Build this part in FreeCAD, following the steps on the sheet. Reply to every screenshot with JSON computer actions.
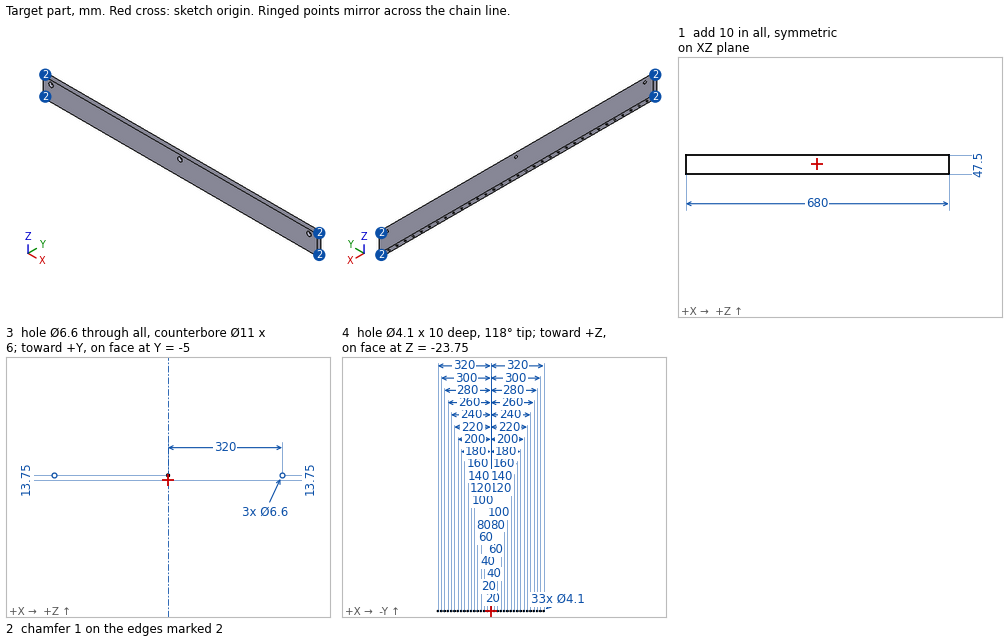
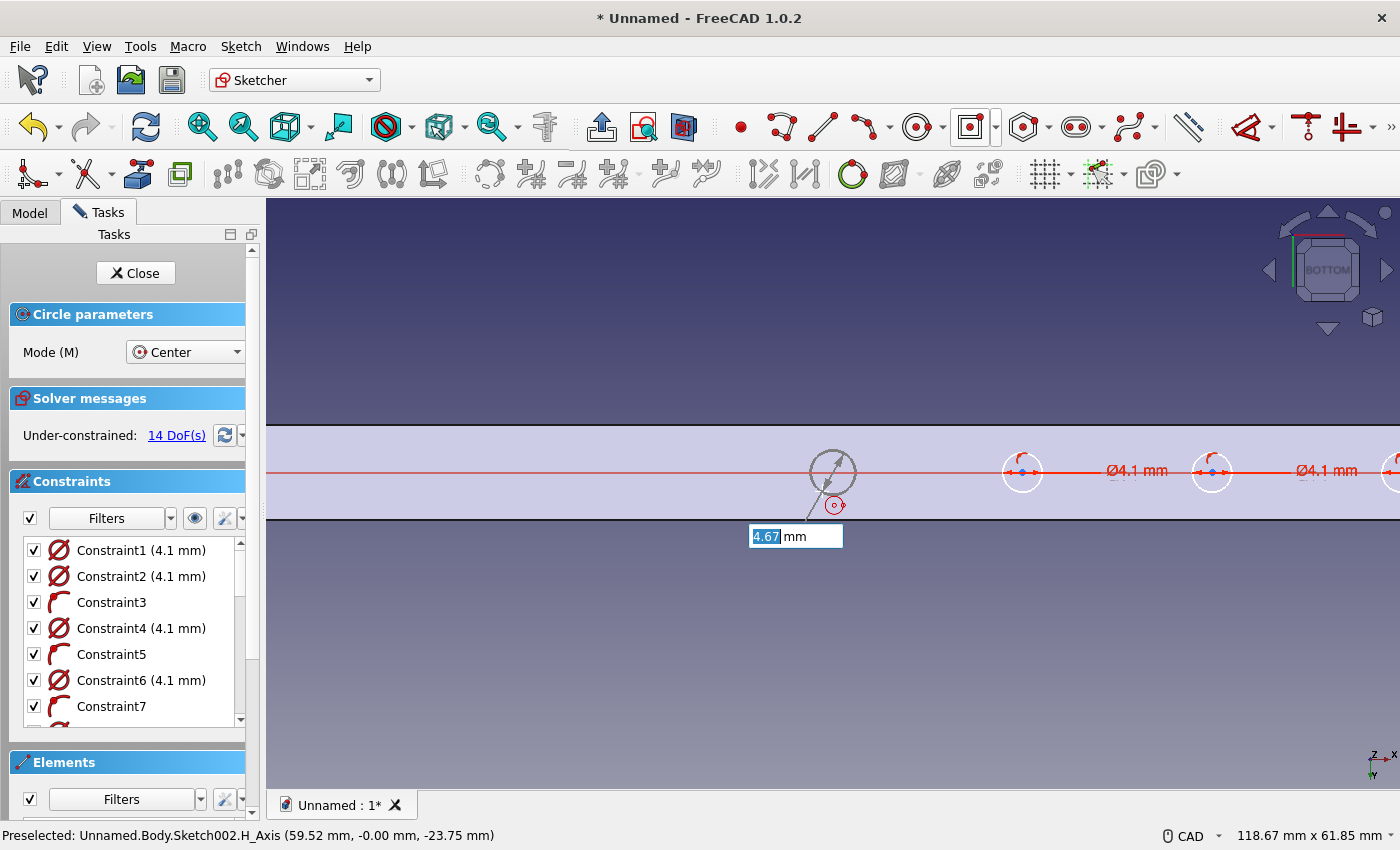
{"action": "type", "text": "4.1"}
{"action": "key", "text": "Return"}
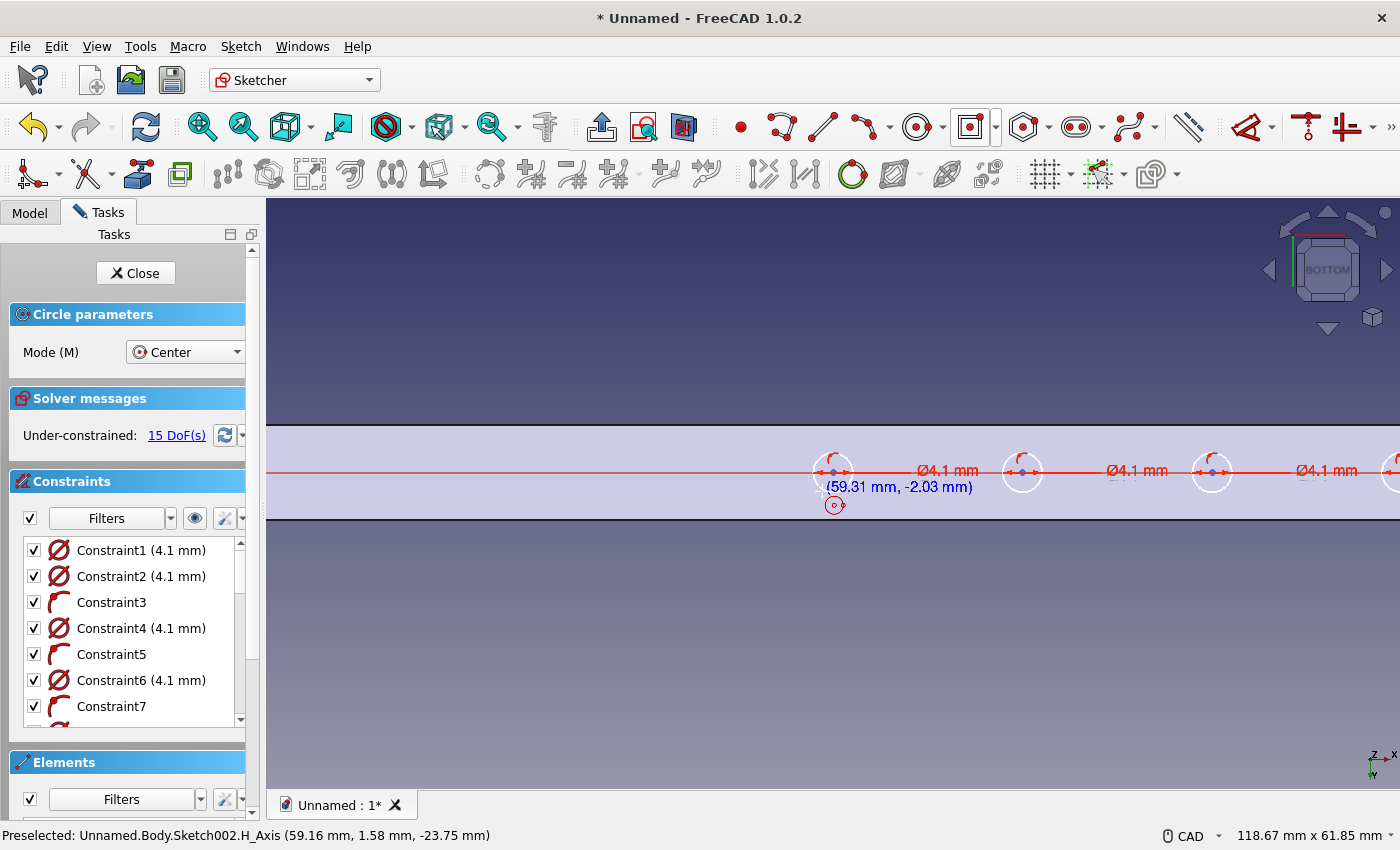
{"action": "scroll", "coordinate": [828, 496], "scroll_direction": "down", "scroll_amount": 11}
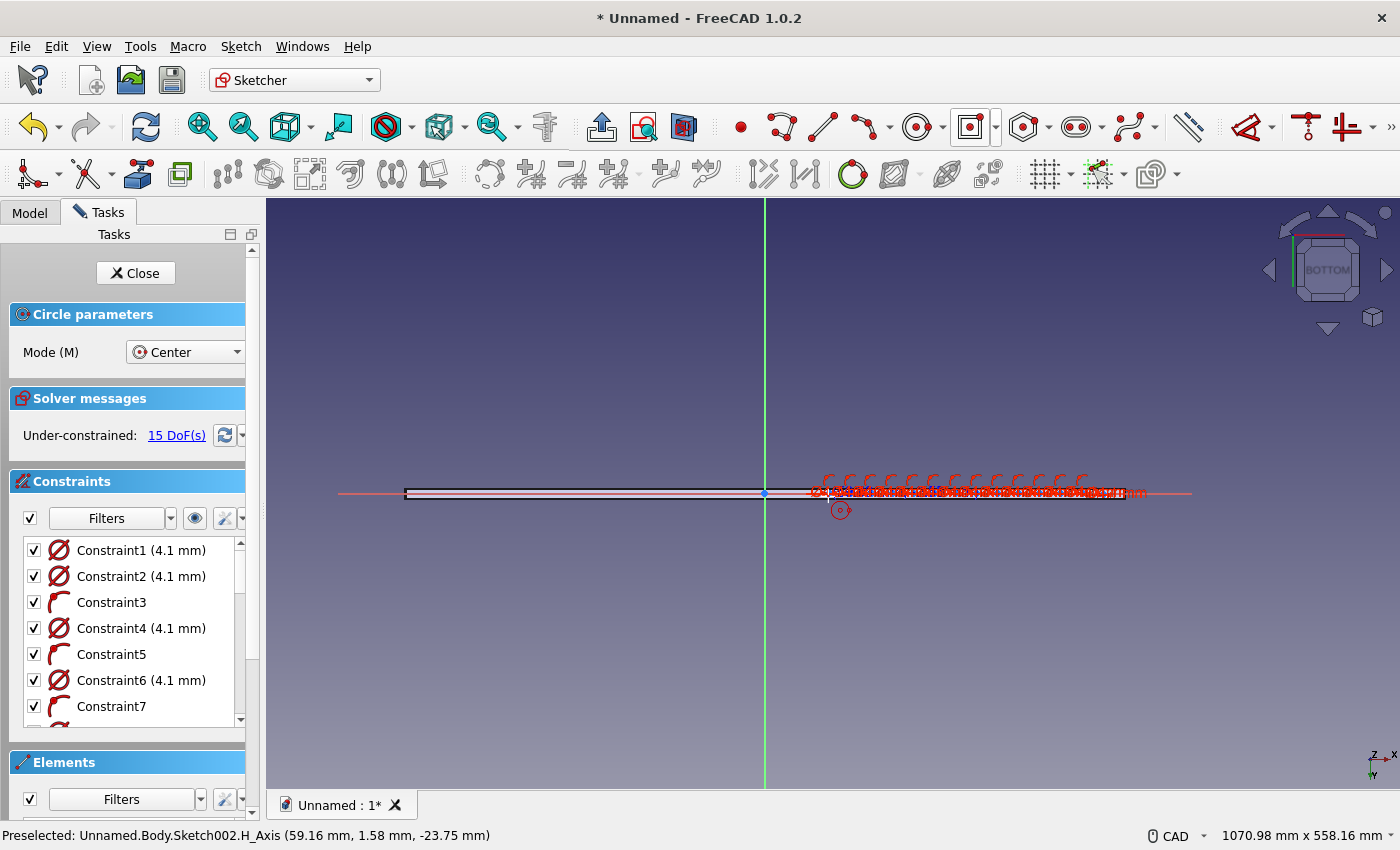
{"action": "left_click", "coordinate": [807, 494]}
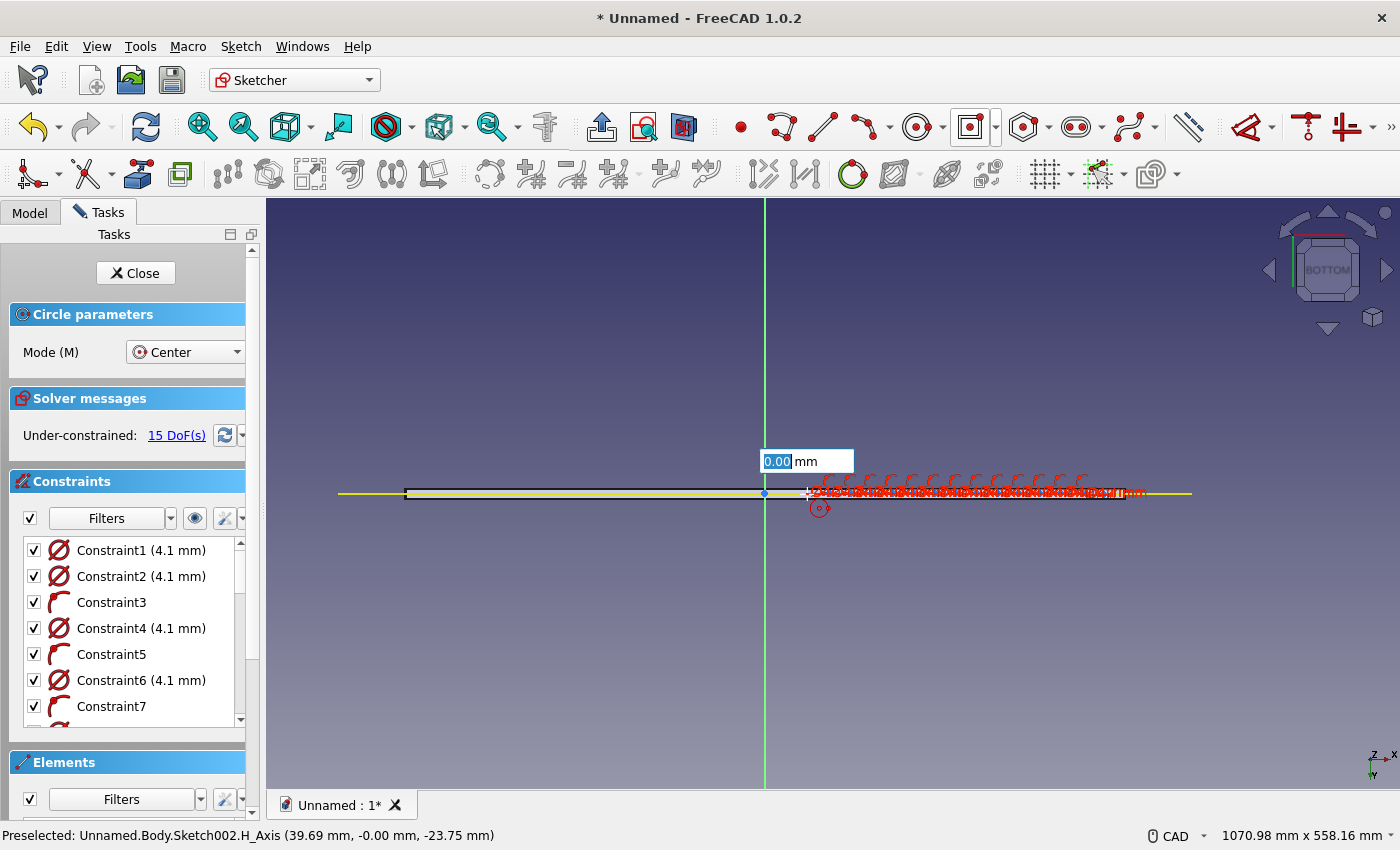
{"action": "scroll", "coordinate": [808, 492], "scroll_direction": "up", "scroll_amount": 11}
{"action": "mouse_move", "coordinate": [805, 486]}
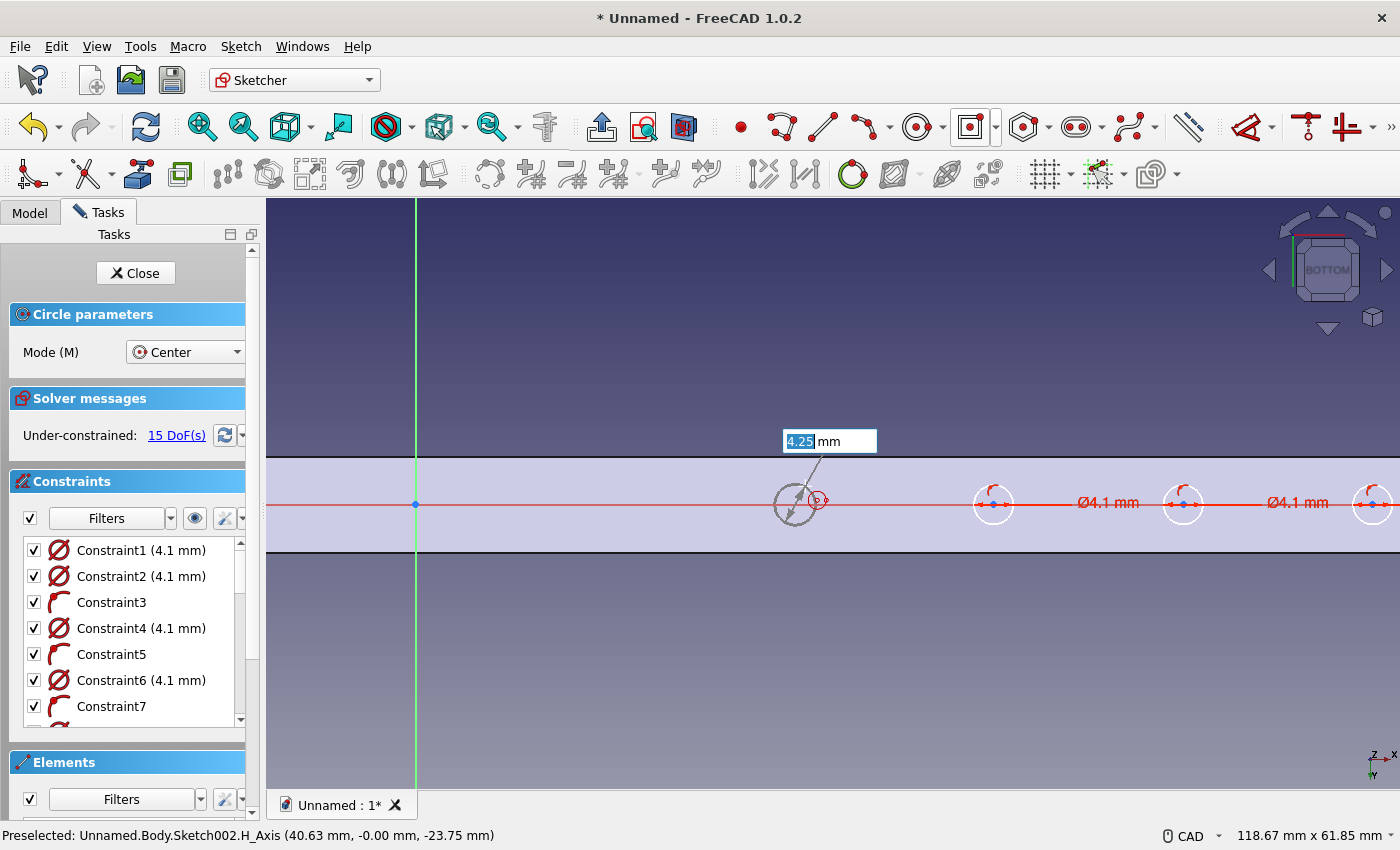
{"action": "type", "text": "4.1"}
{"action": "key", "text": "Return"}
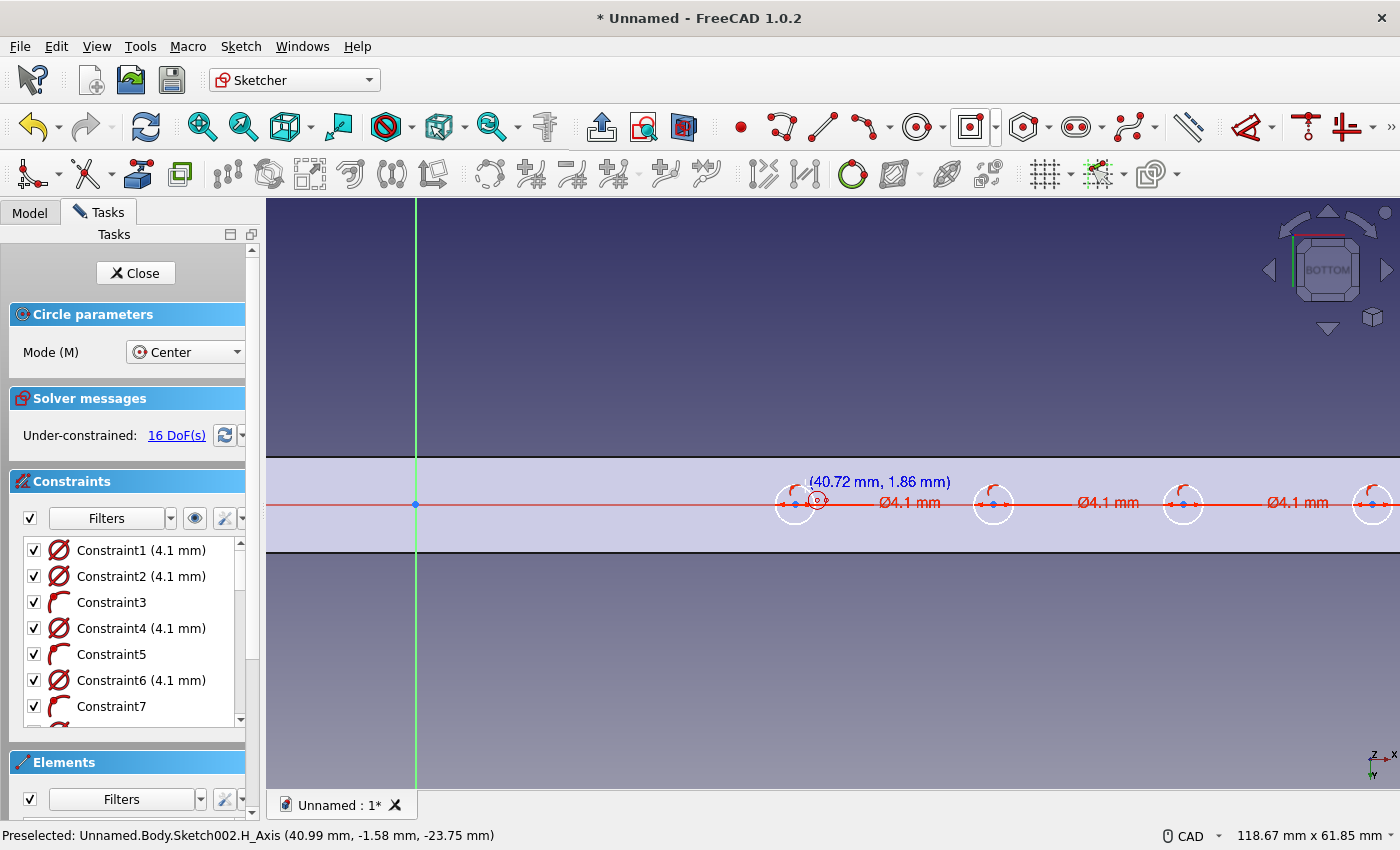
{"action": "scroll", "coordinate": [808, 492], "scroll_direction": "down", "scroll_amount": 11}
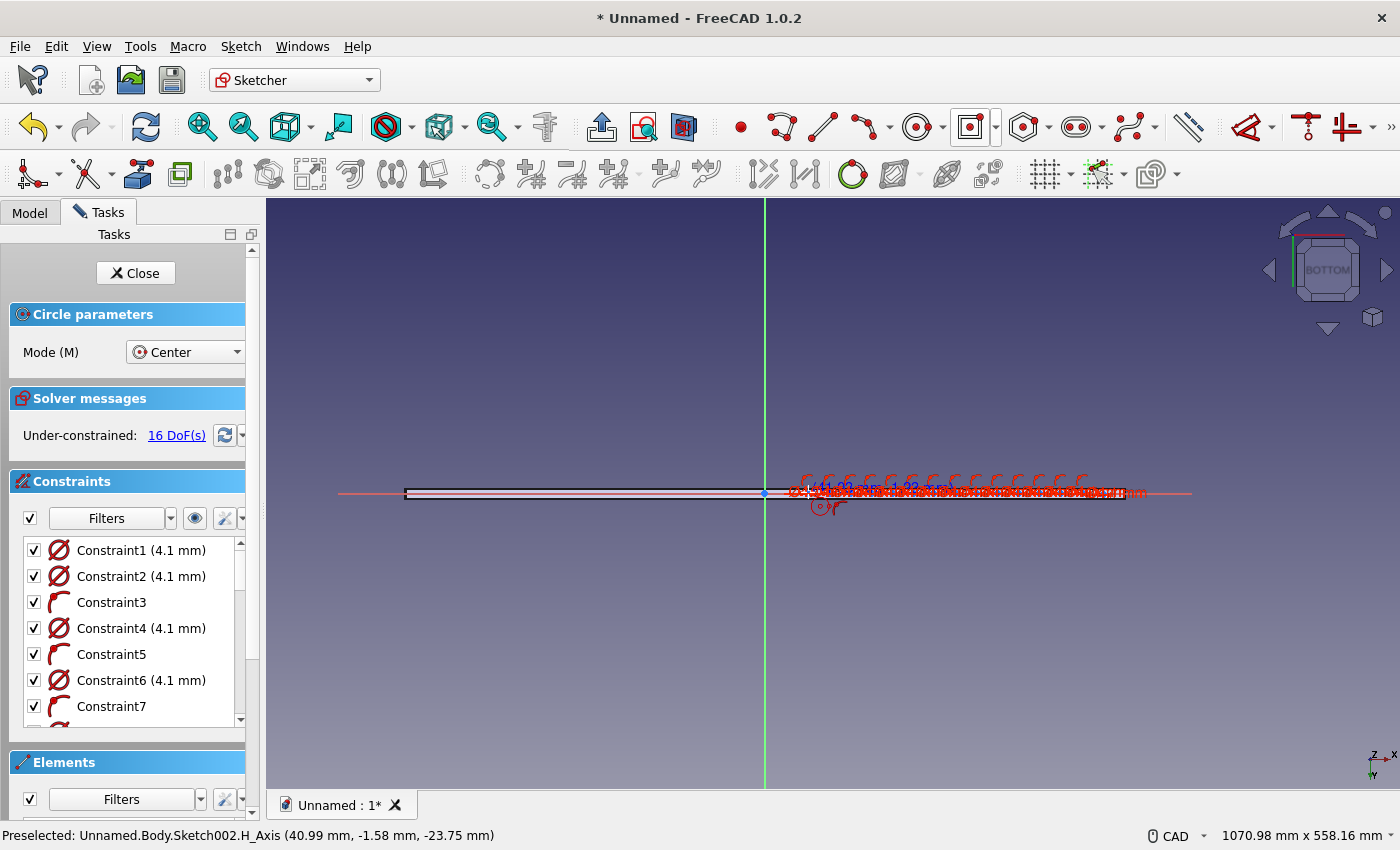
{"action": "left_click", "coordinate": [786, 494]}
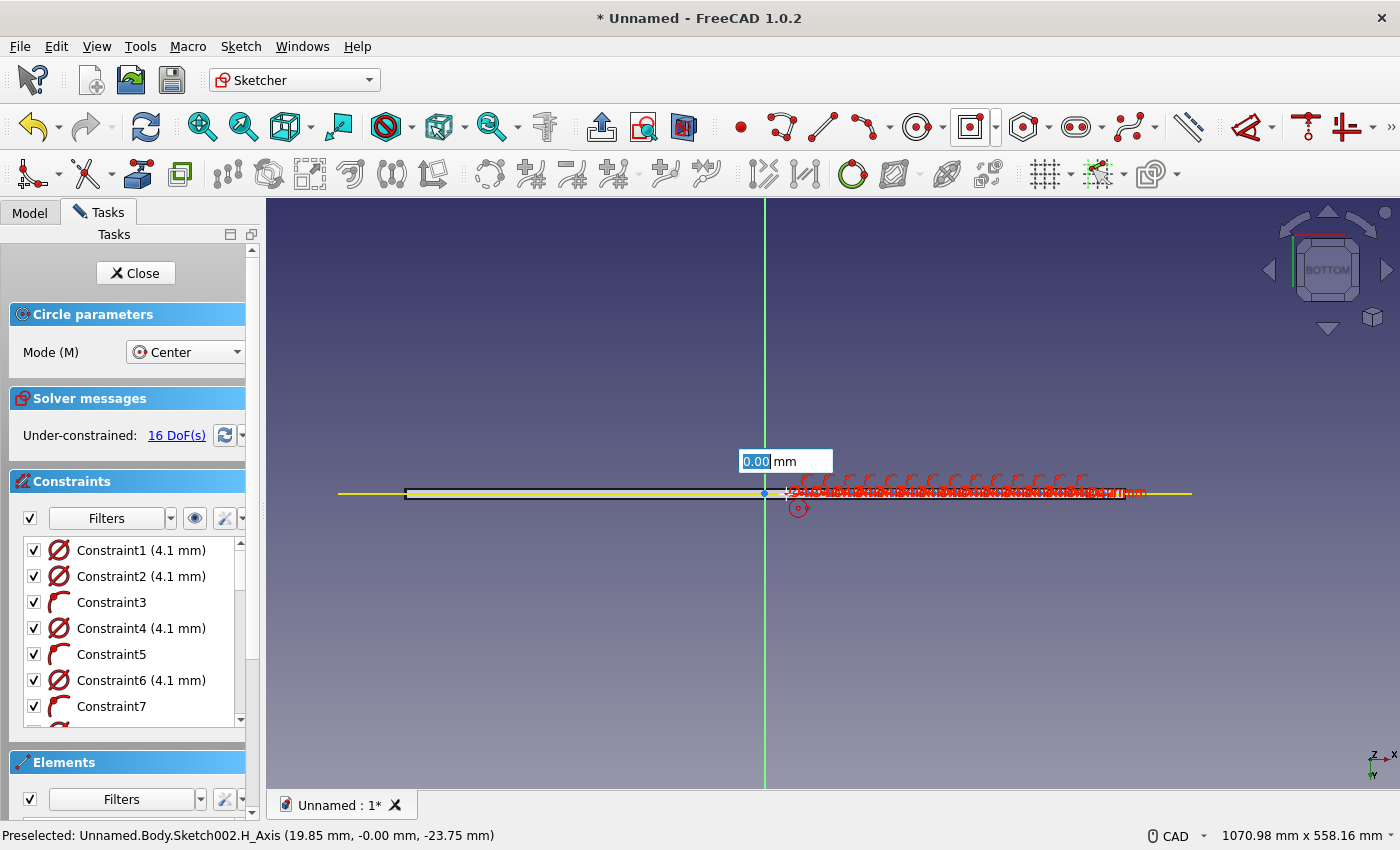
{"action": "scroll", "coordinate": [787, 492], "scroll_direction": "up", "scroll_amount": 11}
{"action": "mouse_move", "coordinate": [782, 486]}